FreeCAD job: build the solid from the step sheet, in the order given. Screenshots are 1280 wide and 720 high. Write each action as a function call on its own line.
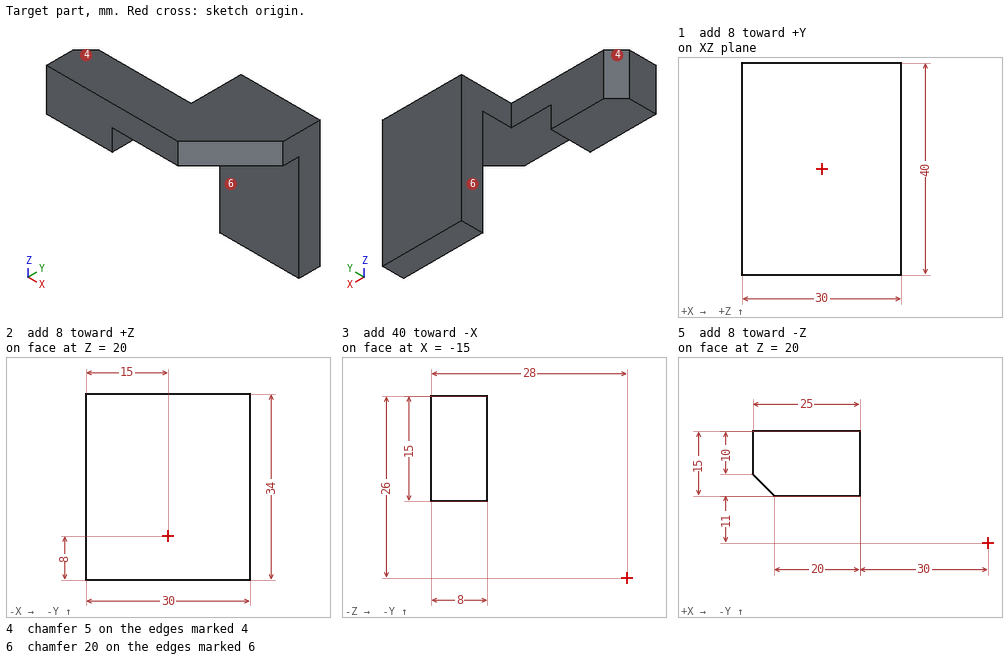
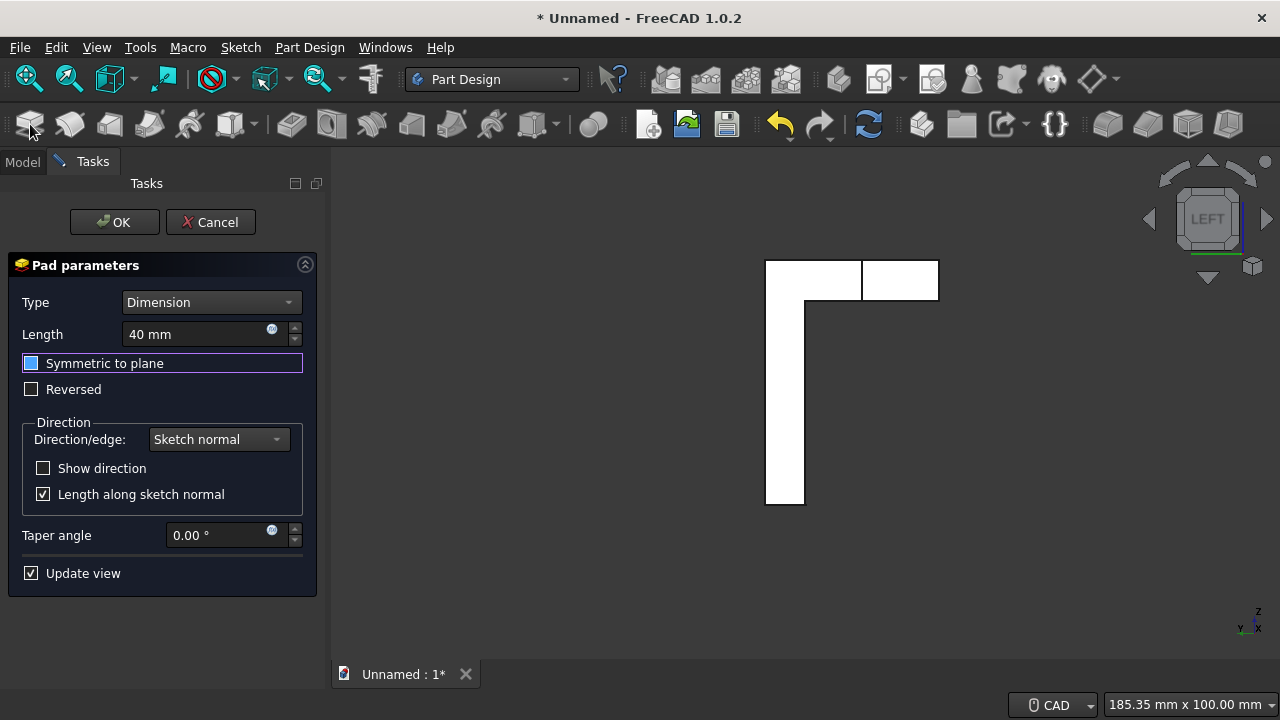
click(115, 222)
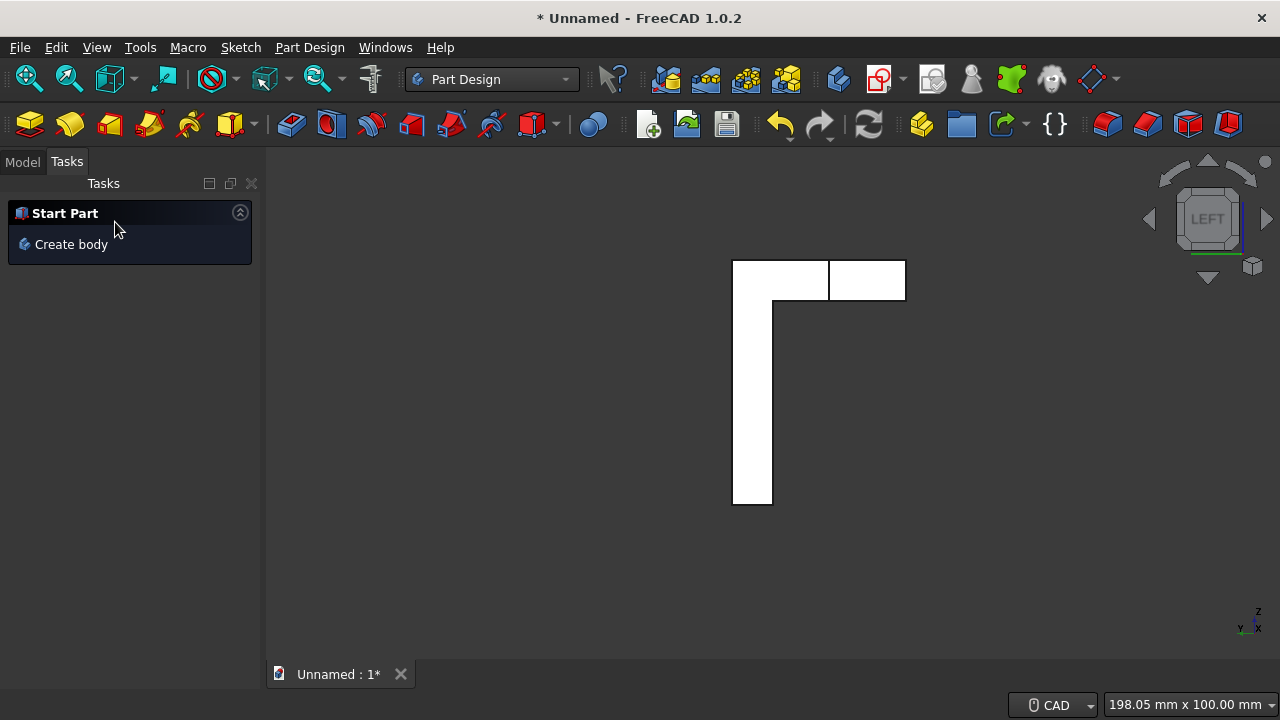
click(829, 279)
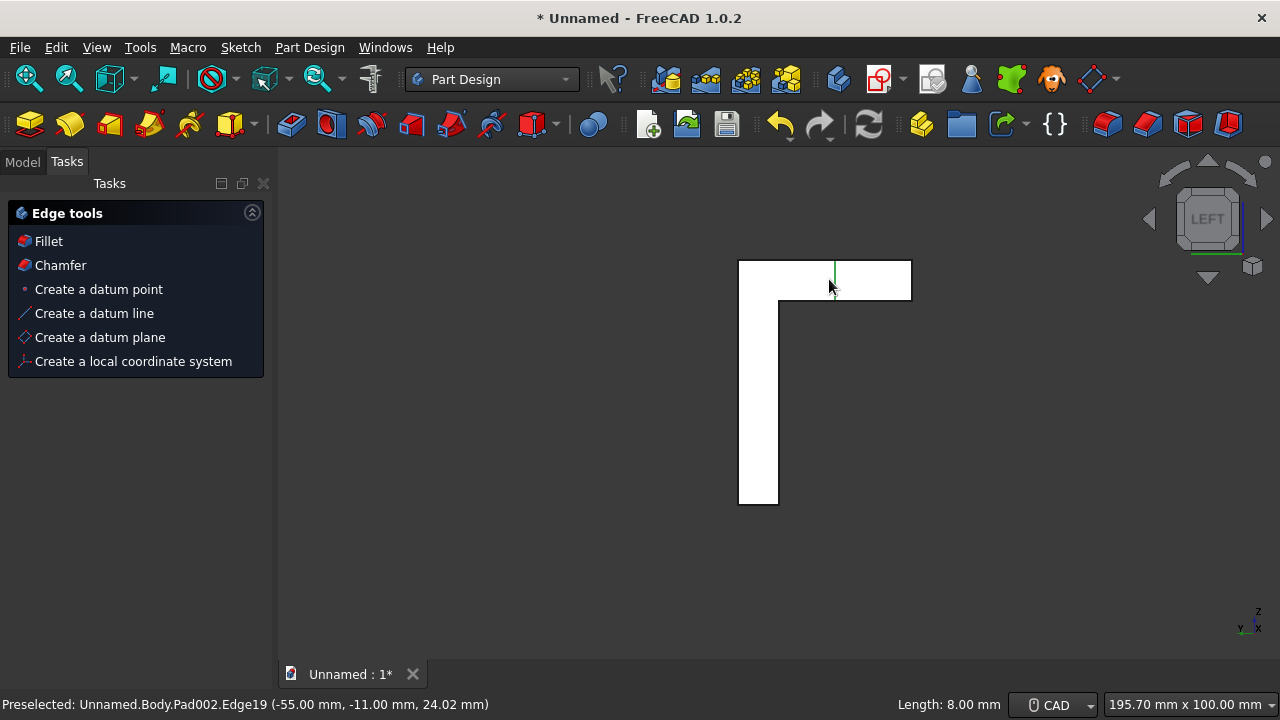
click(1148, 124)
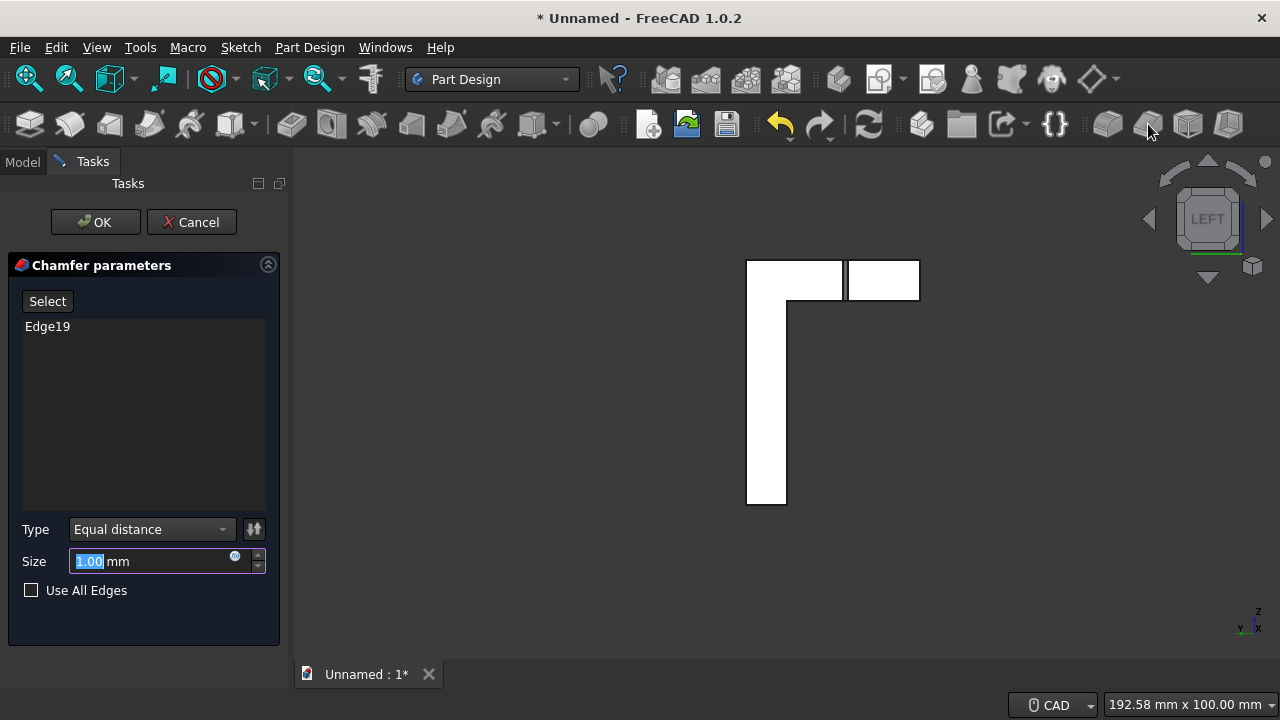
text(5)
key(Tab)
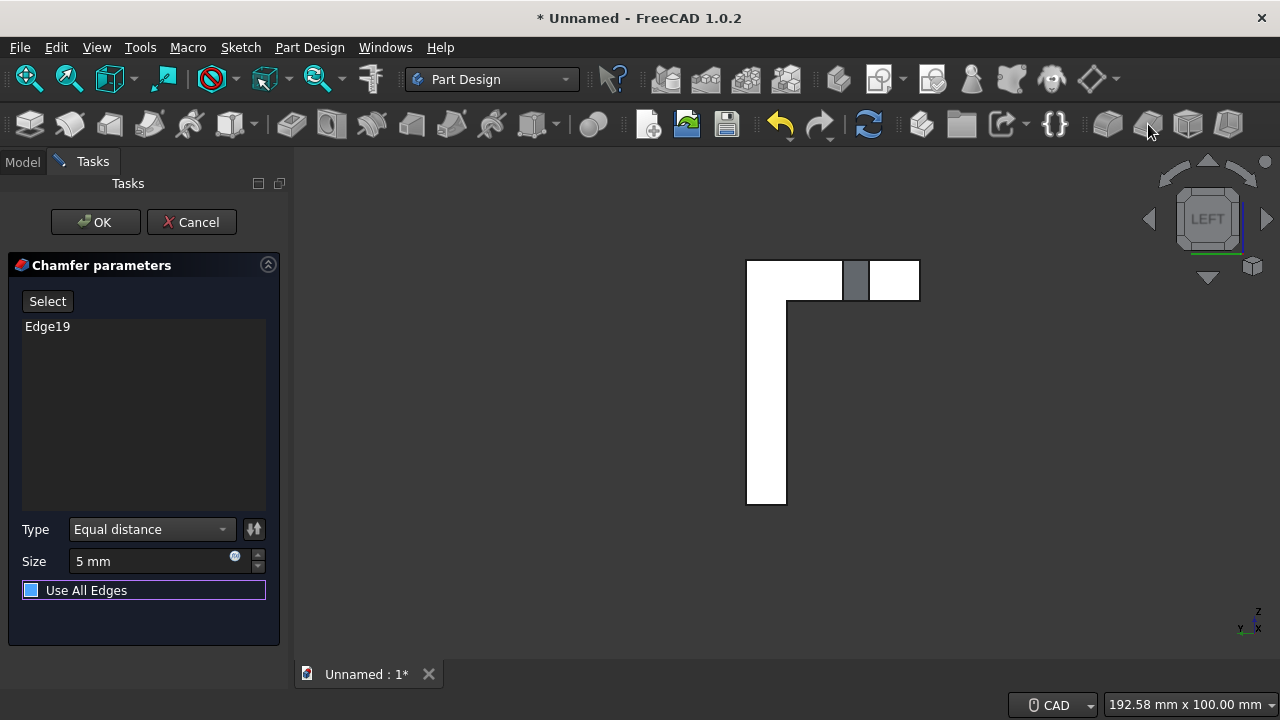
click(96, 222)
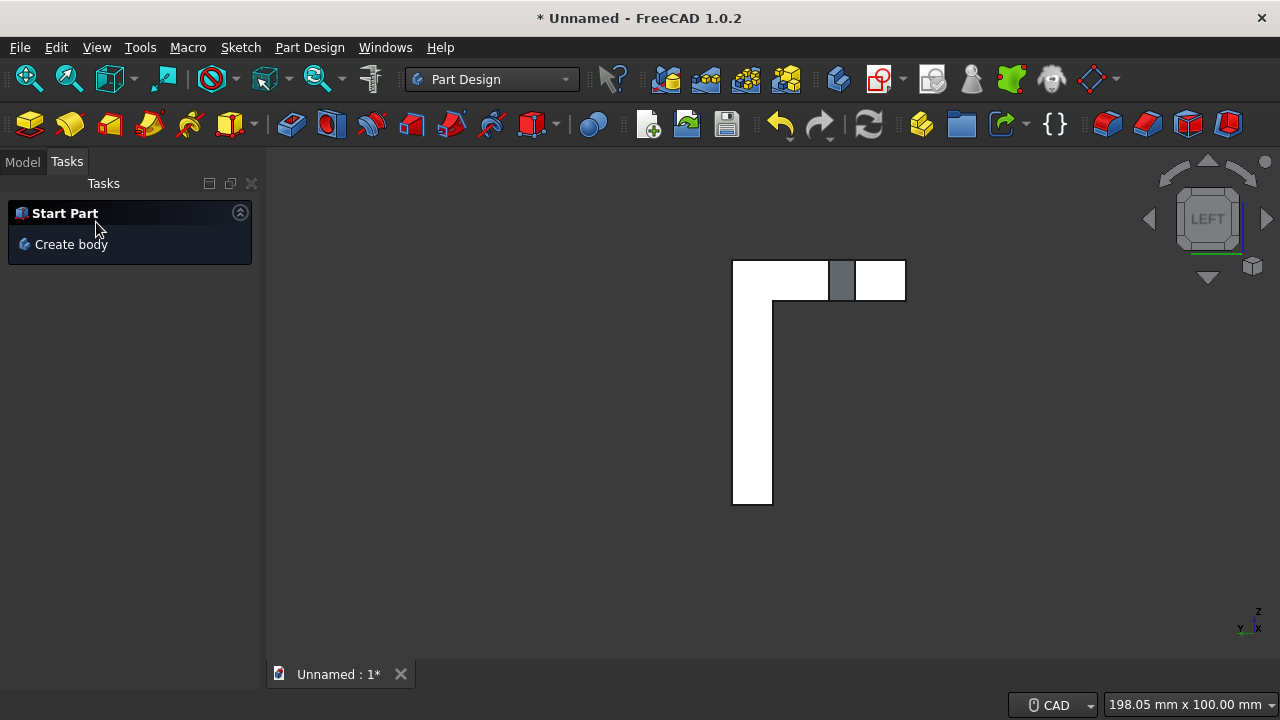
key(5)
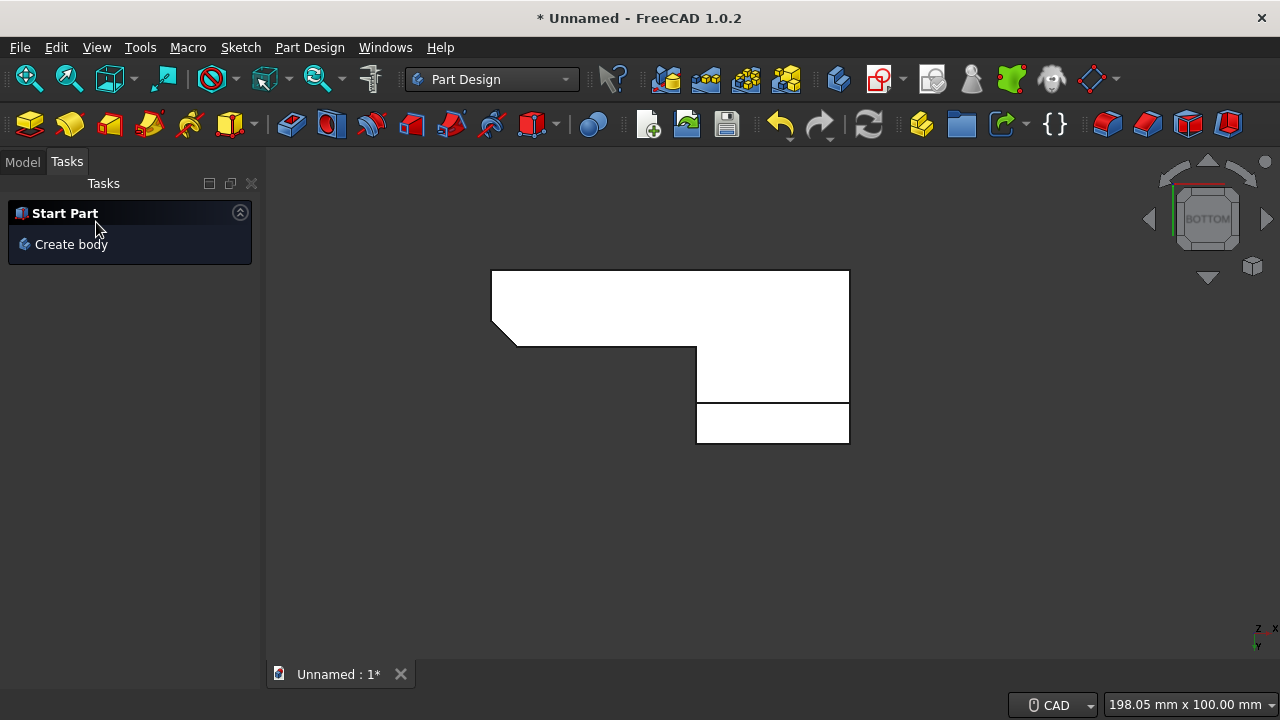
click(30, 80)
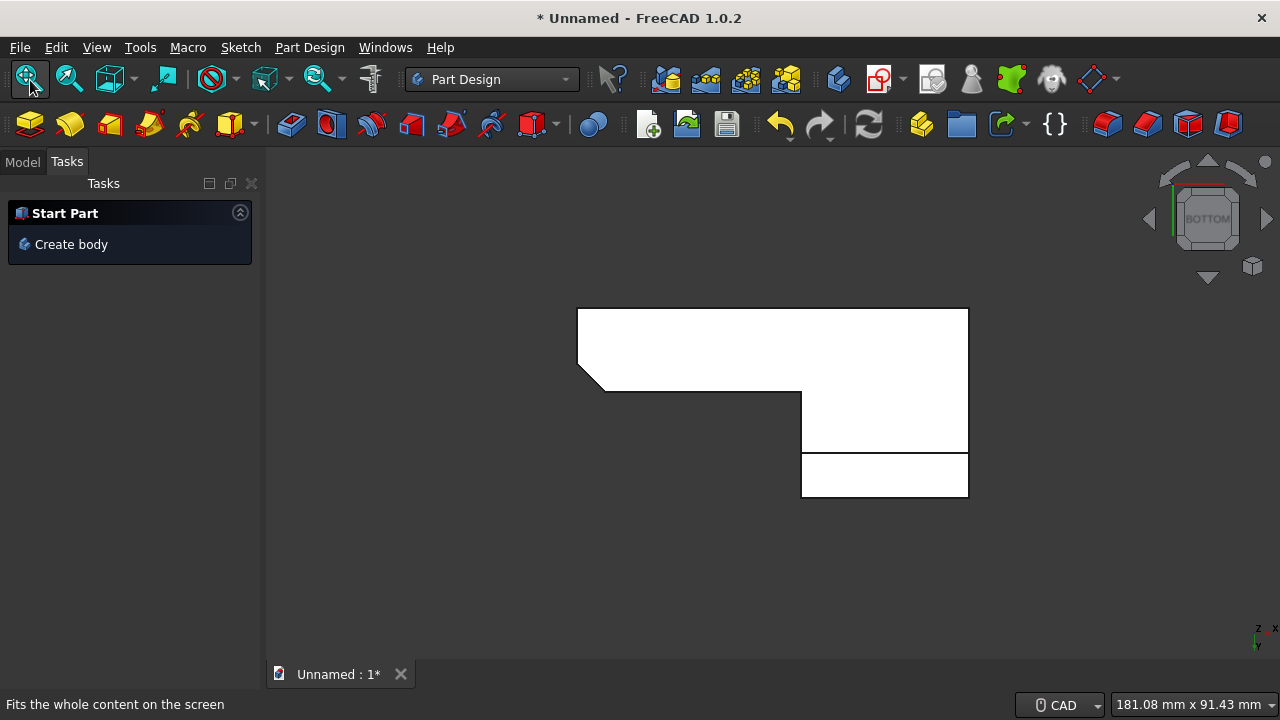
click(885, 380)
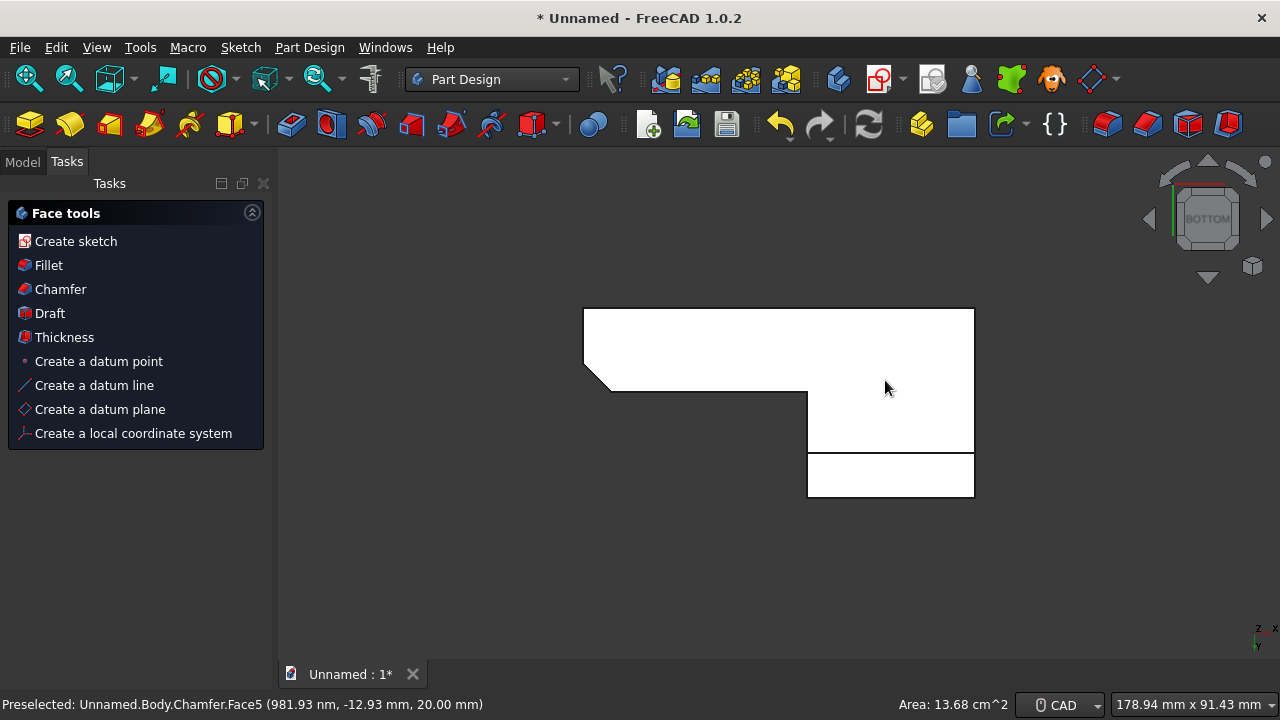
click(880, 80)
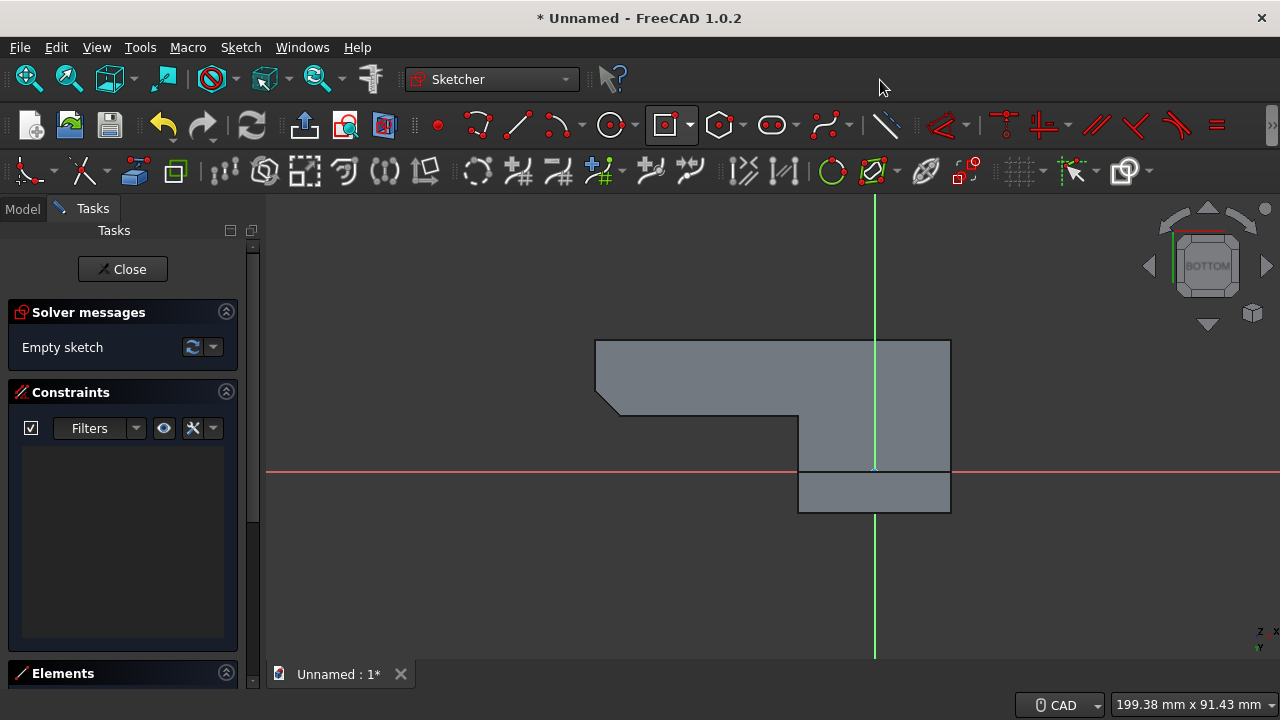
scroll(760, 390, up, 4)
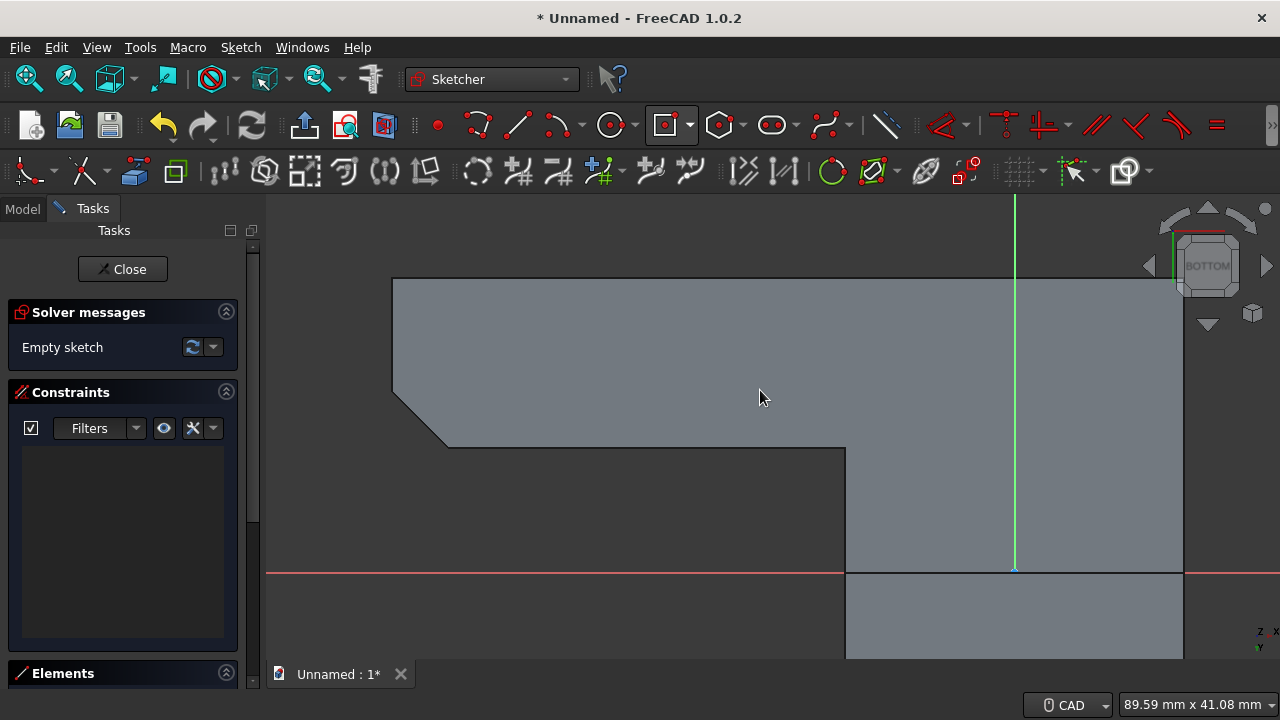
click(478, 126)